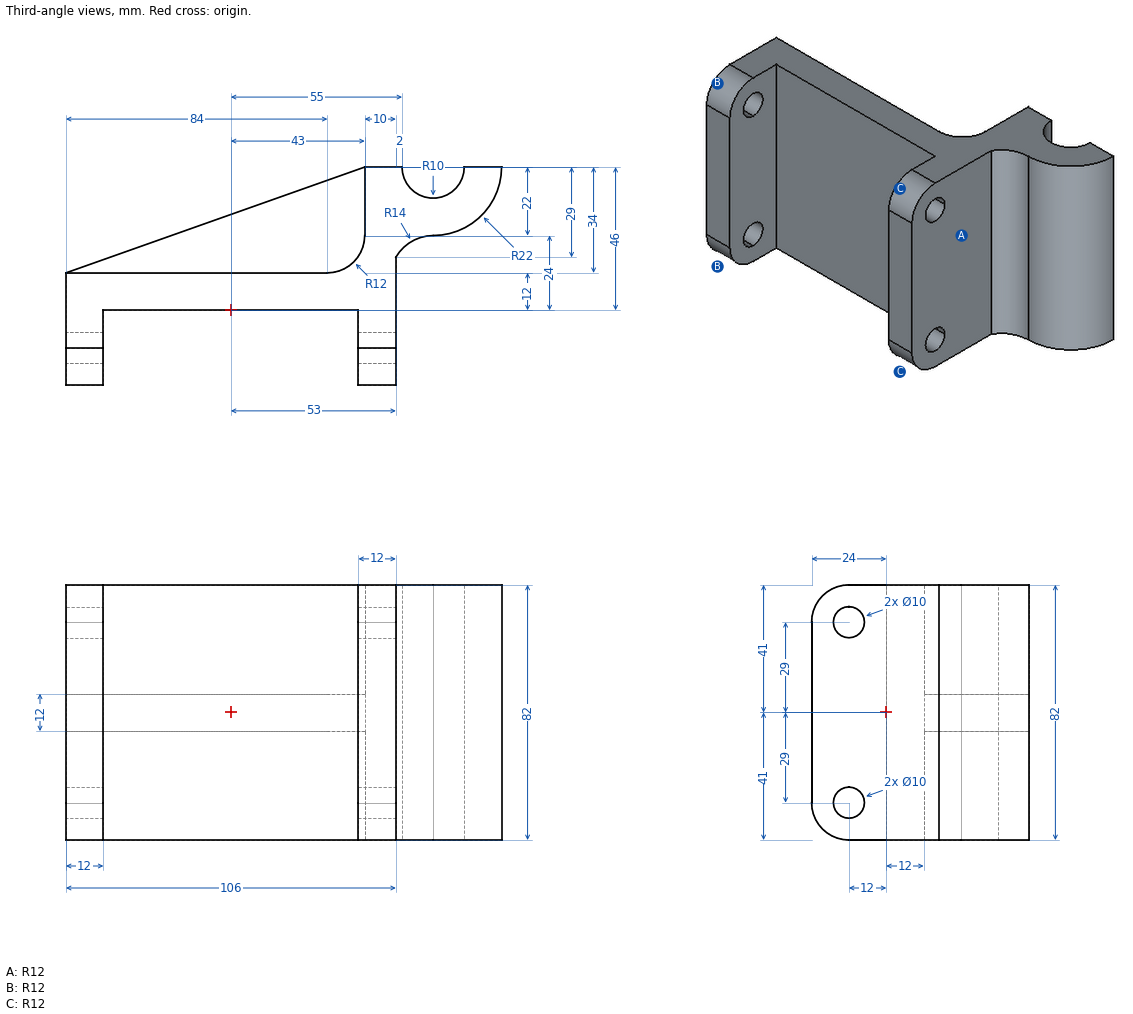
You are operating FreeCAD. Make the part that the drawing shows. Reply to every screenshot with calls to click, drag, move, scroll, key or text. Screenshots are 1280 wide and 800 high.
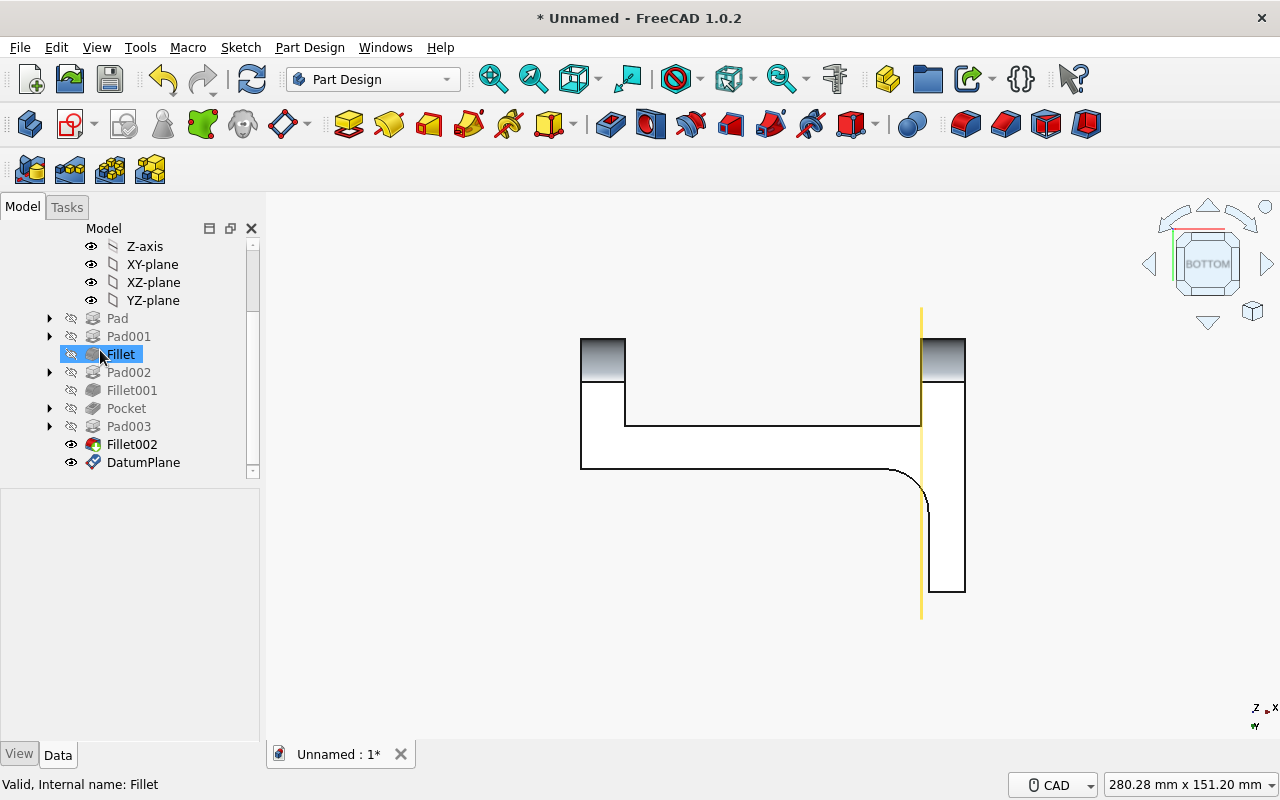
click(116, 462)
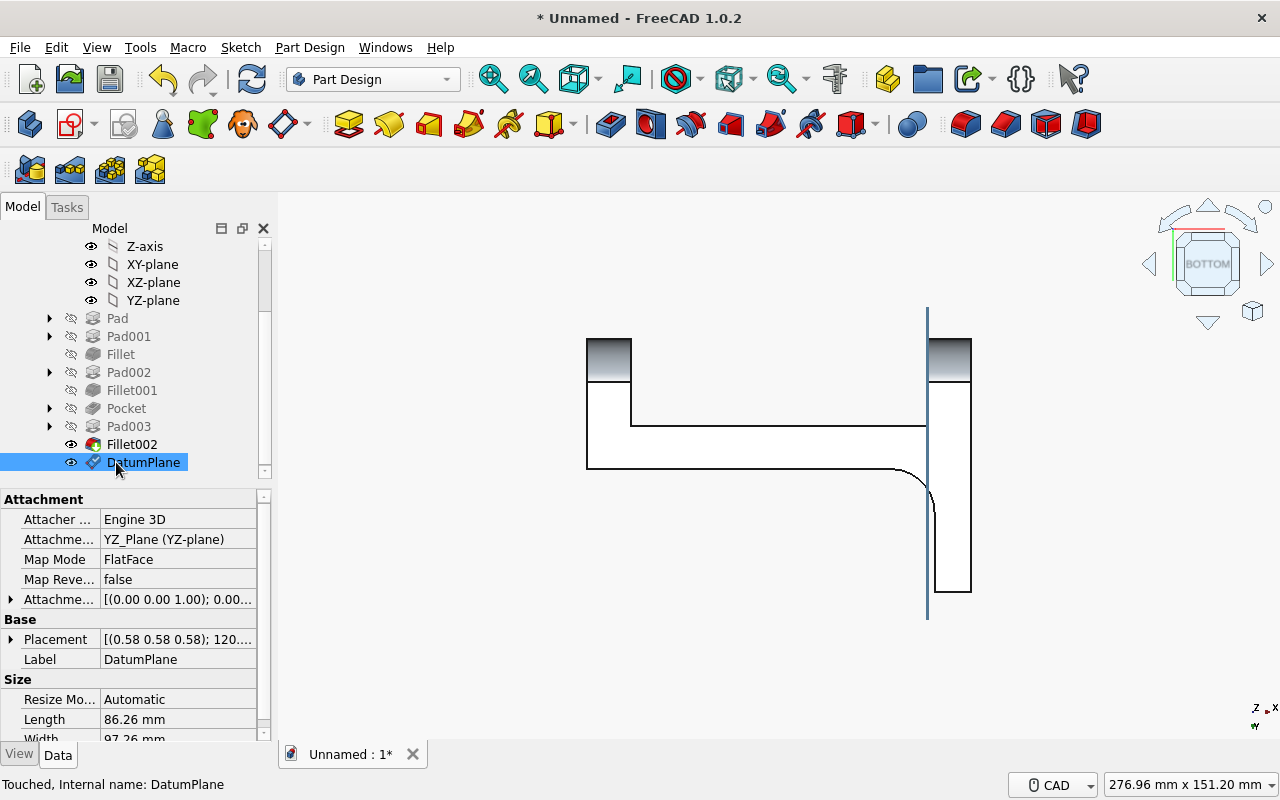
click(70, 124)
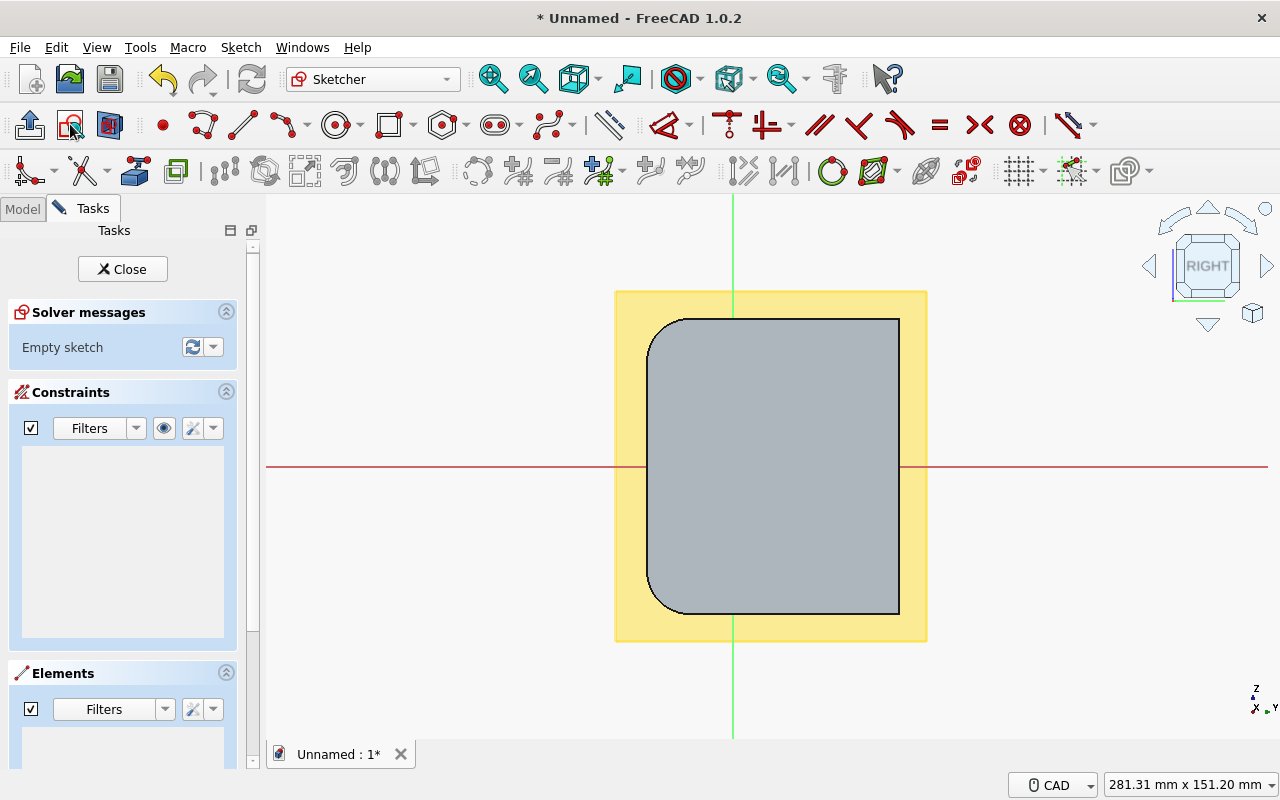
key(q)
key(s)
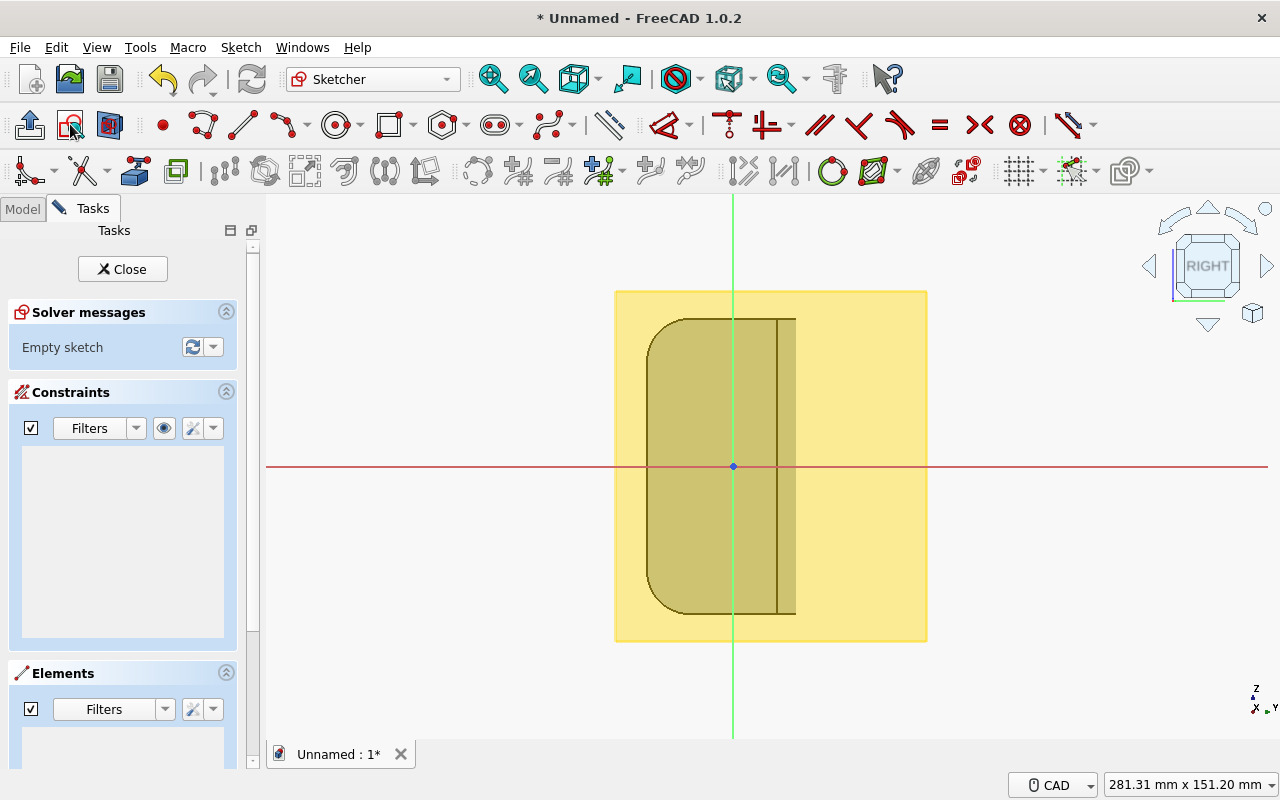
scroll(699, 467, up, 2)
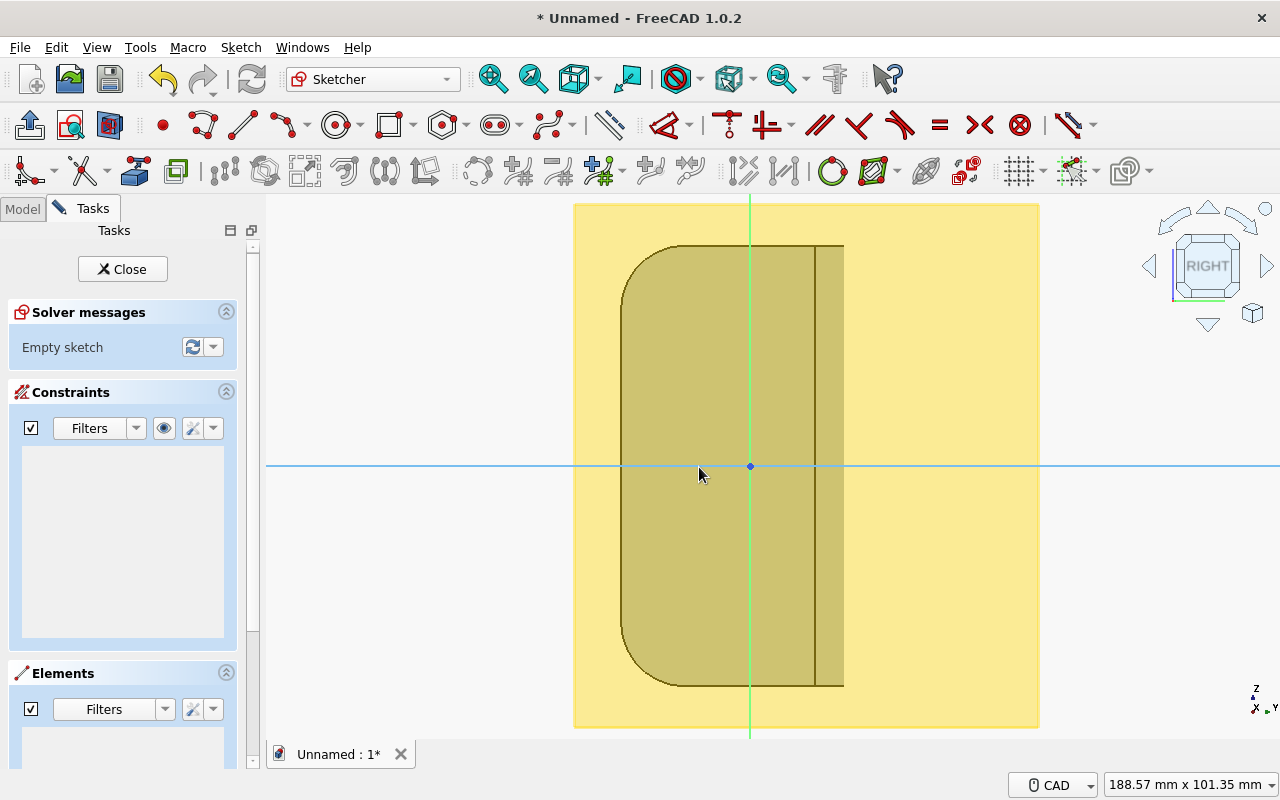
click(336, 126)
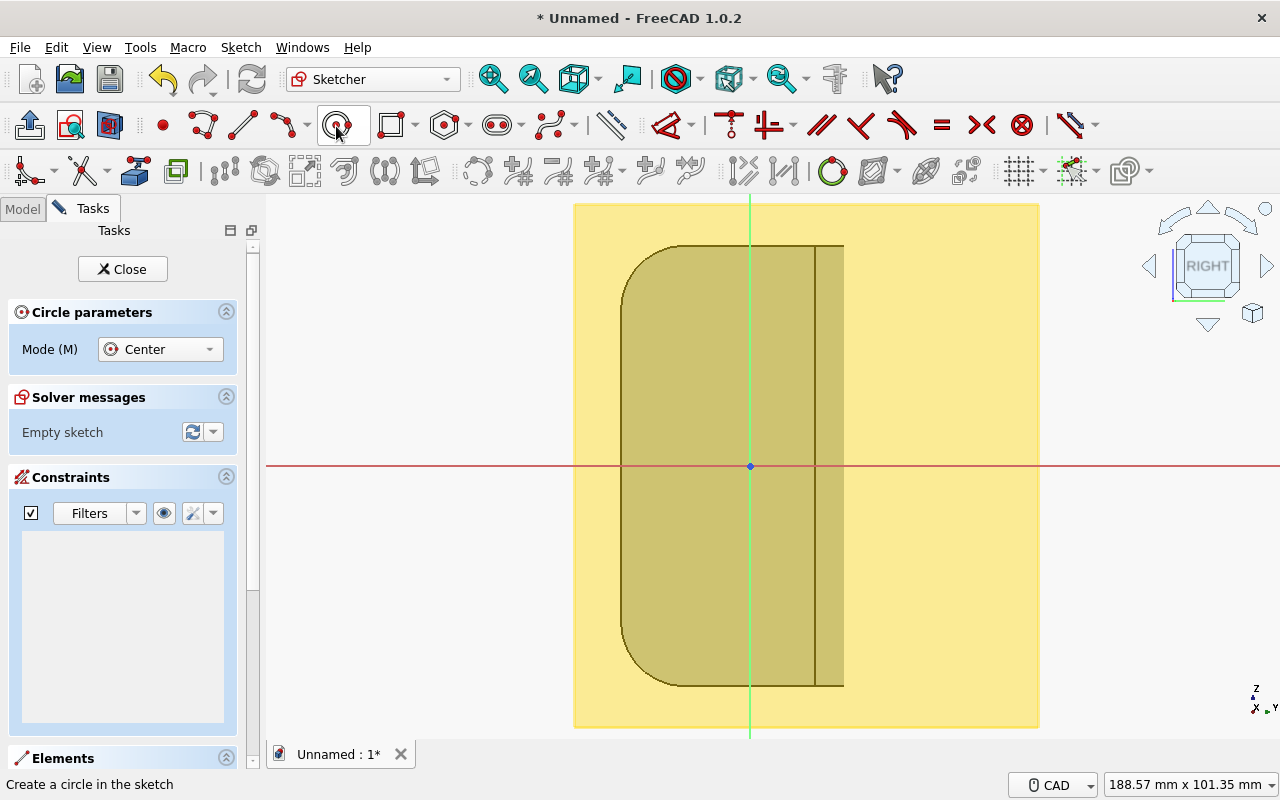
click(686, 310)
move(705, 291)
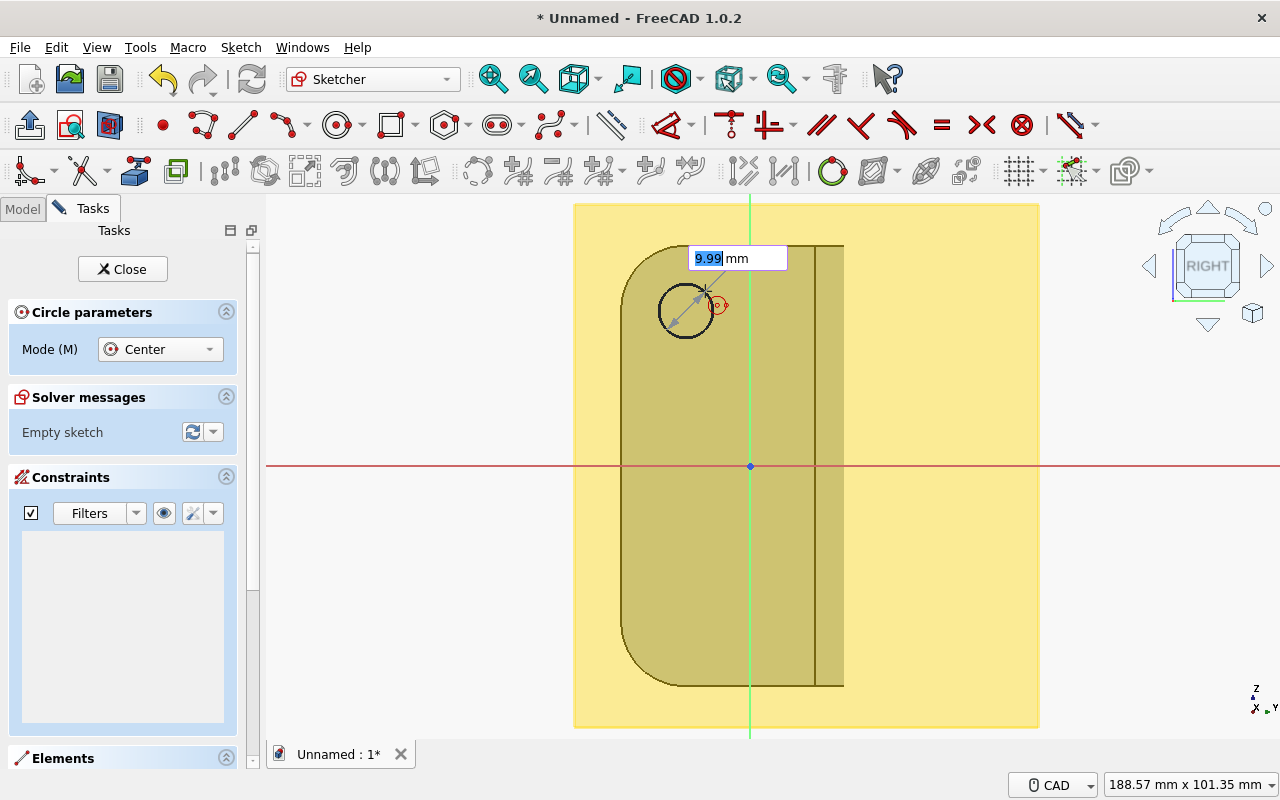
text(10)
key(Return)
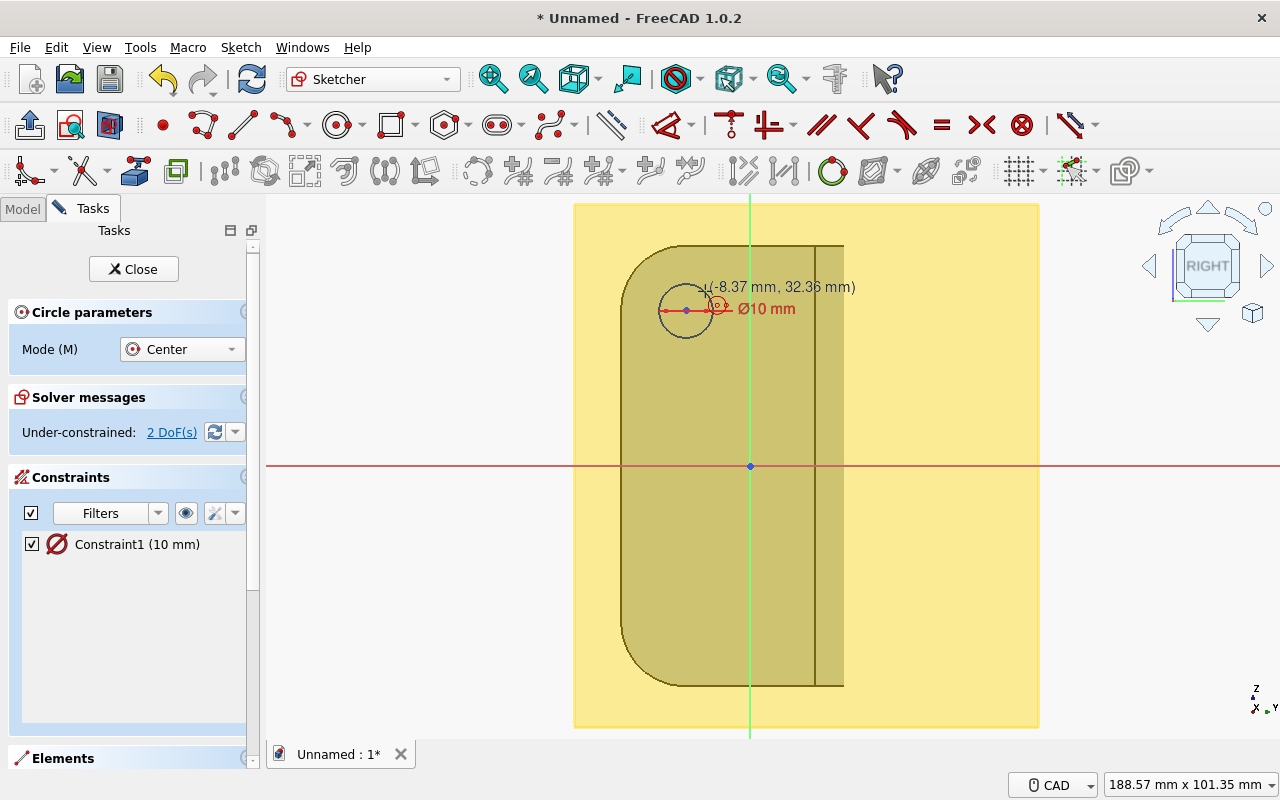
click(686, 622)
move(705, 603)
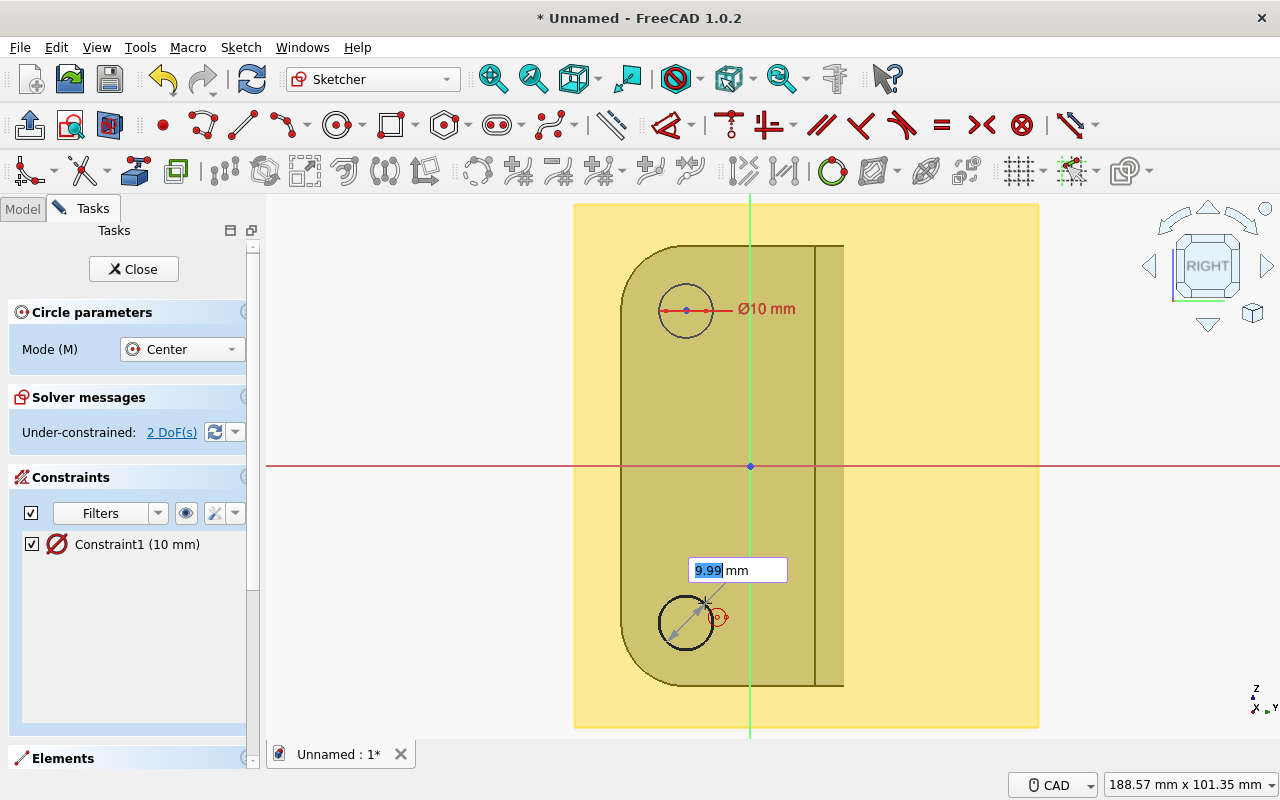
text(10)
key(Return)
key(Escape)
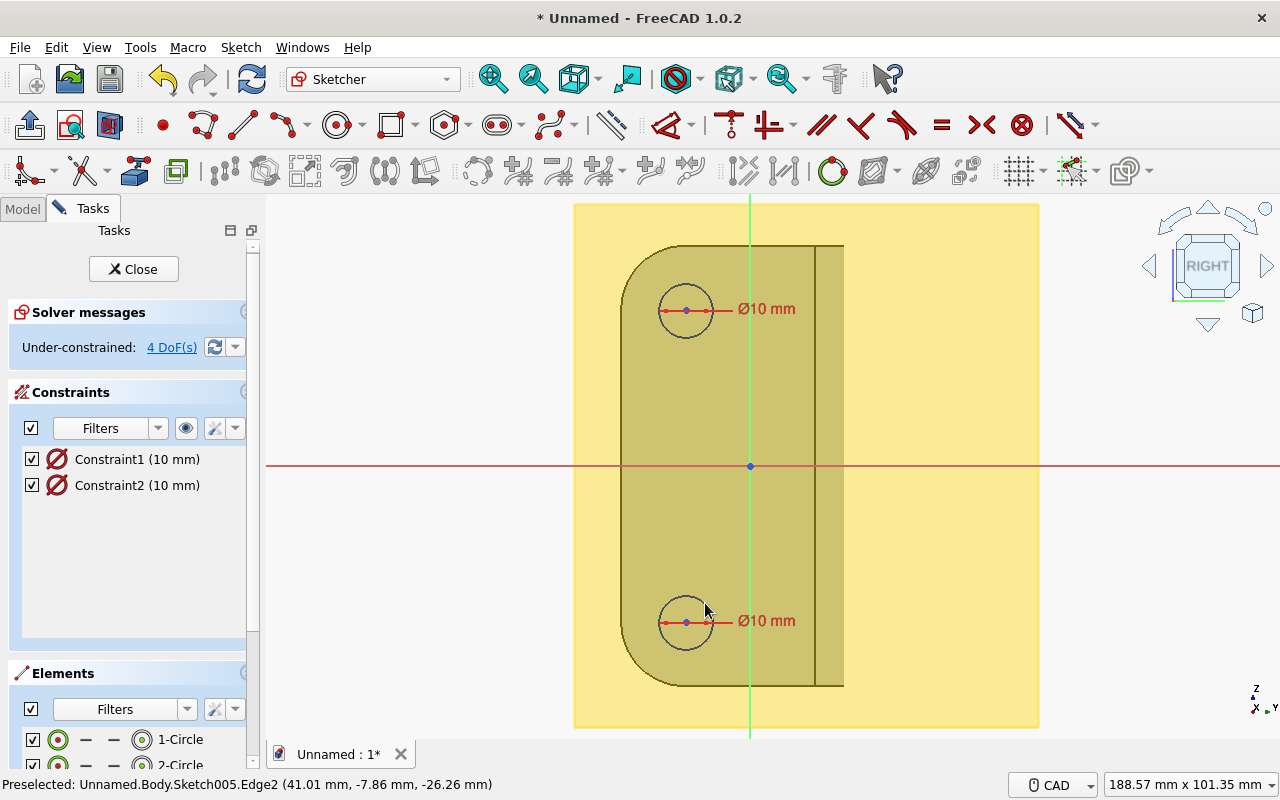
click(686, 311)